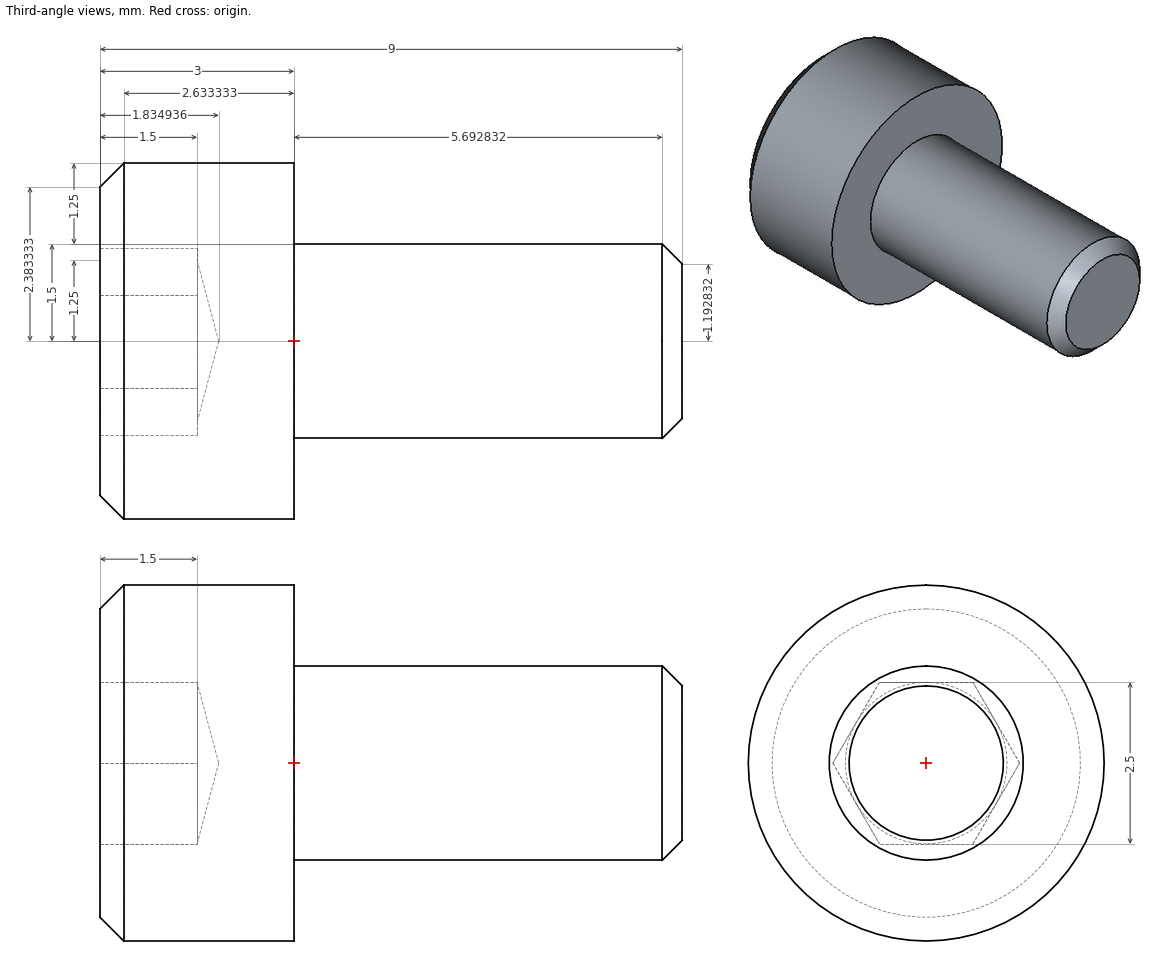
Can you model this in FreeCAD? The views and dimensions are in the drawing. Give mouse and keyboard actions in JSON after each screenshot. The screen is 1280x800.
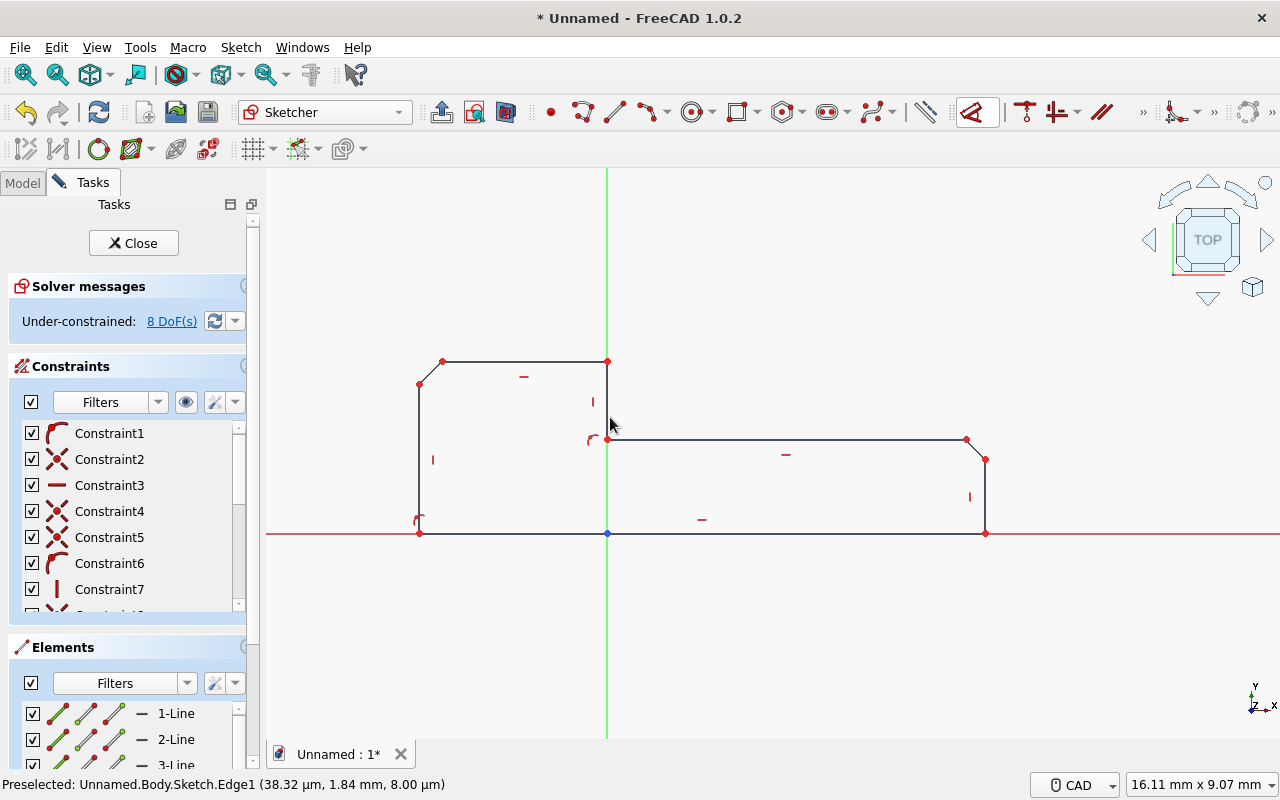
{"action": "left_click", "coordinate": [589, 534]}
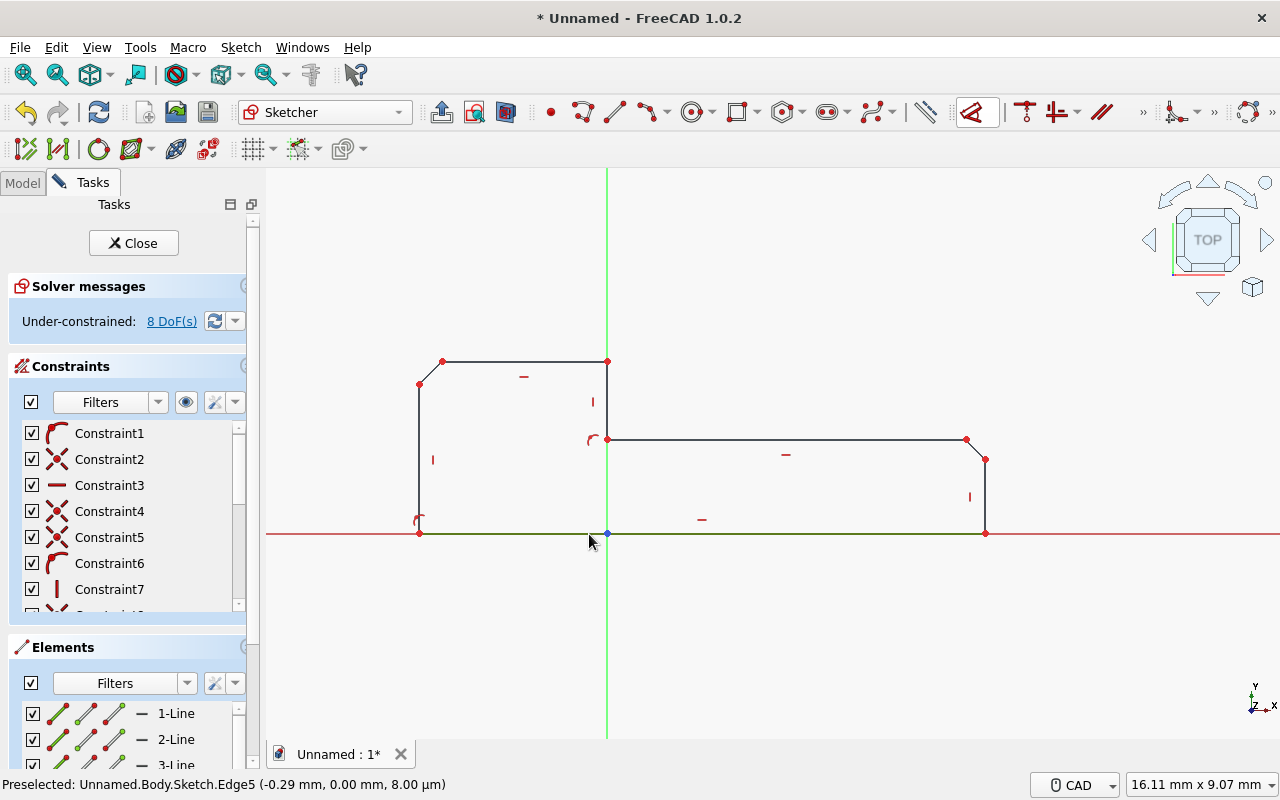
{"action": "left_click", "coordinate": [994, 112]}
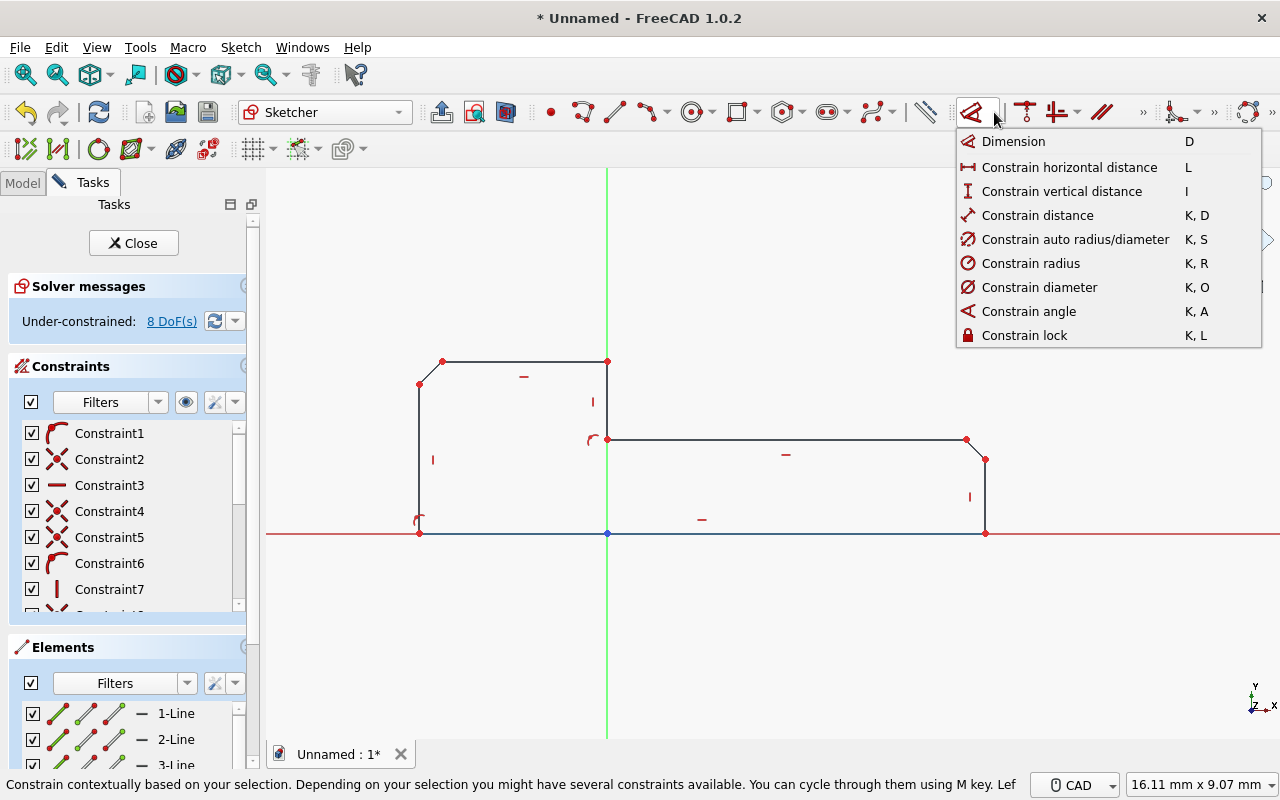
{"action": "left_click", "coordinate": [1109, 167]}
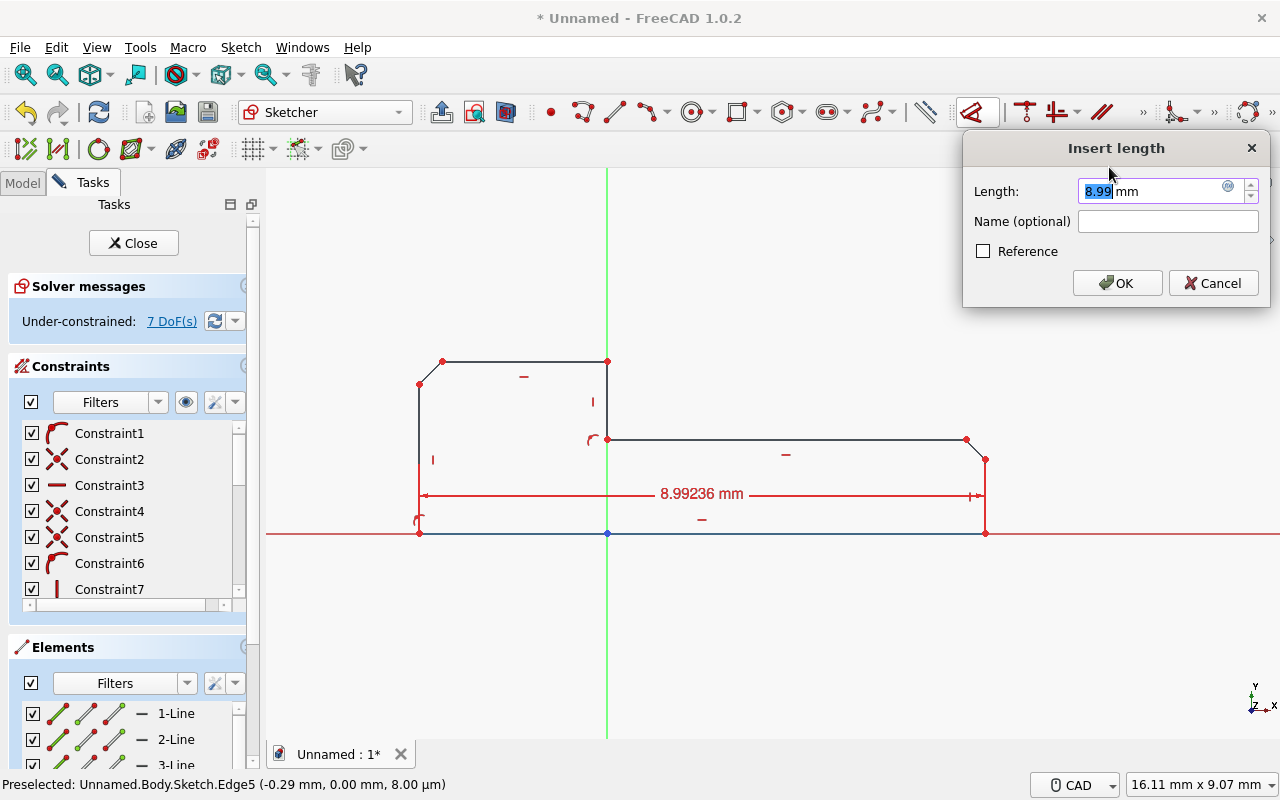
{"action": "type", "text": "9"}
{"action": "key", "text": "Return"}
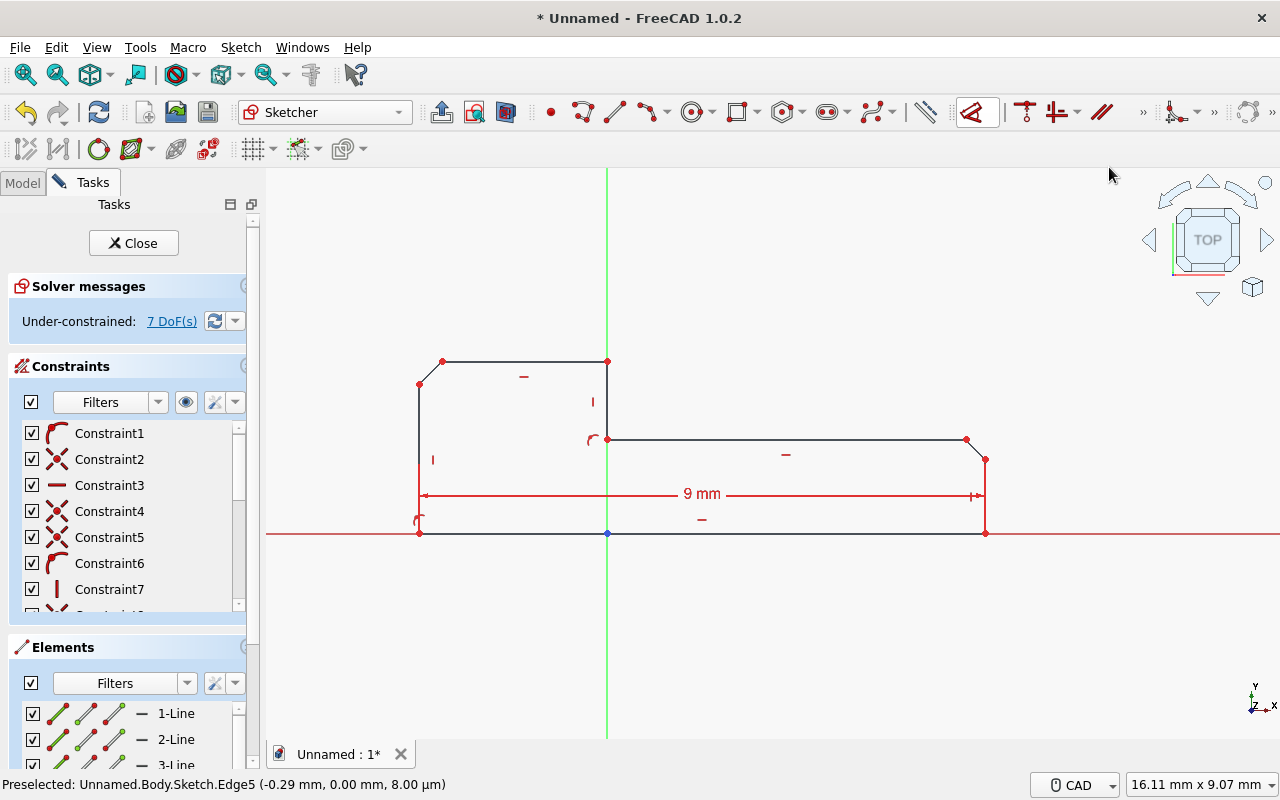
{"action": "left_click", "coordinate": [419, 385]}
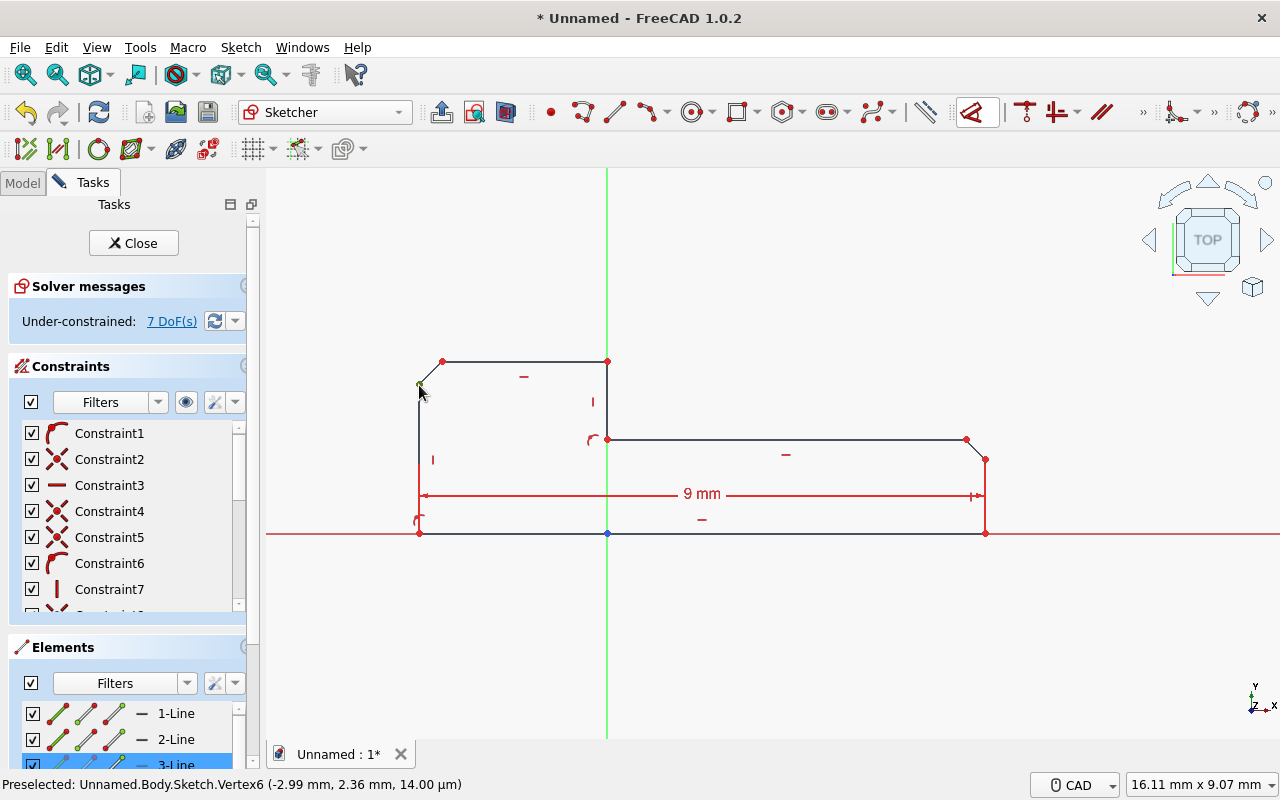
{"action": "left_click", "coordinate": [994, 112]}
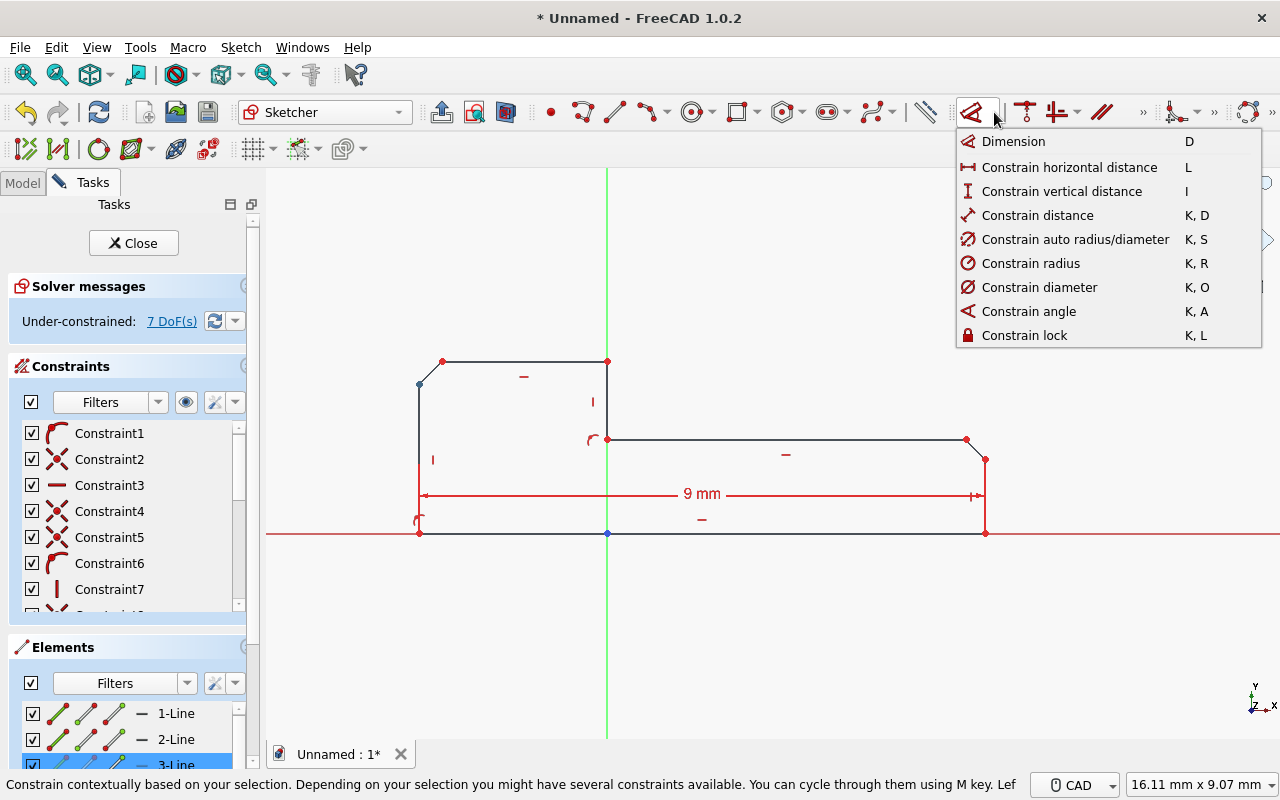
{"action": "left_click", "coordinate": [1109, 167]}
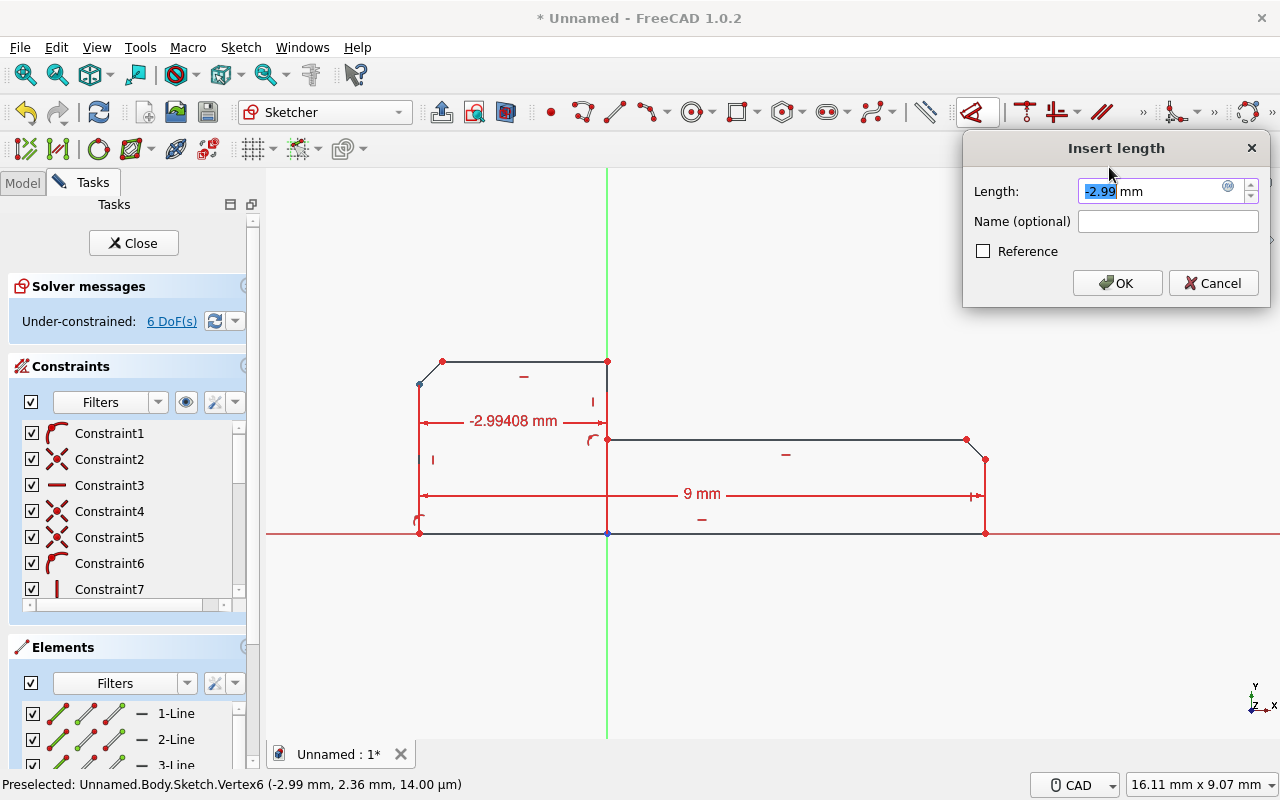
{"action": "type", "text": "-3"}
{"action": "key", "text": "Return"}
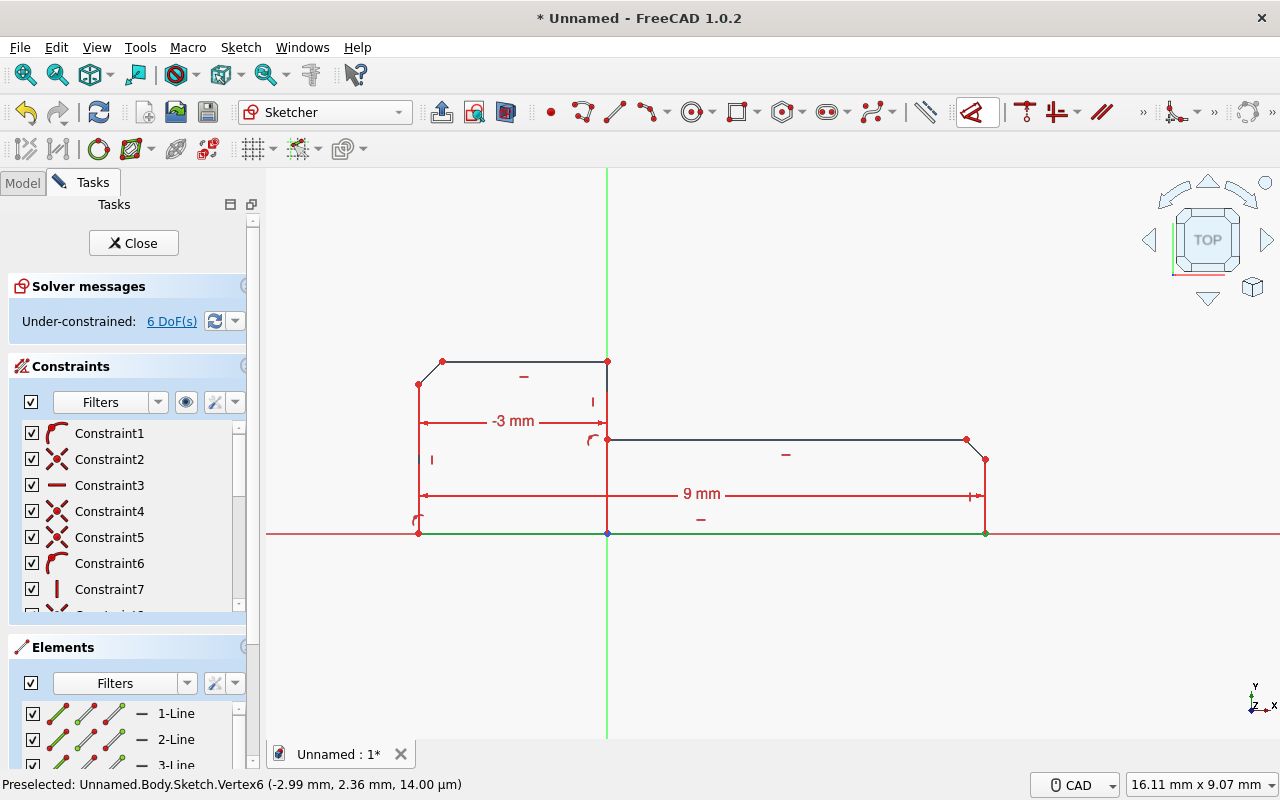
{"action": "left_click", "coordinate": [607, 417]}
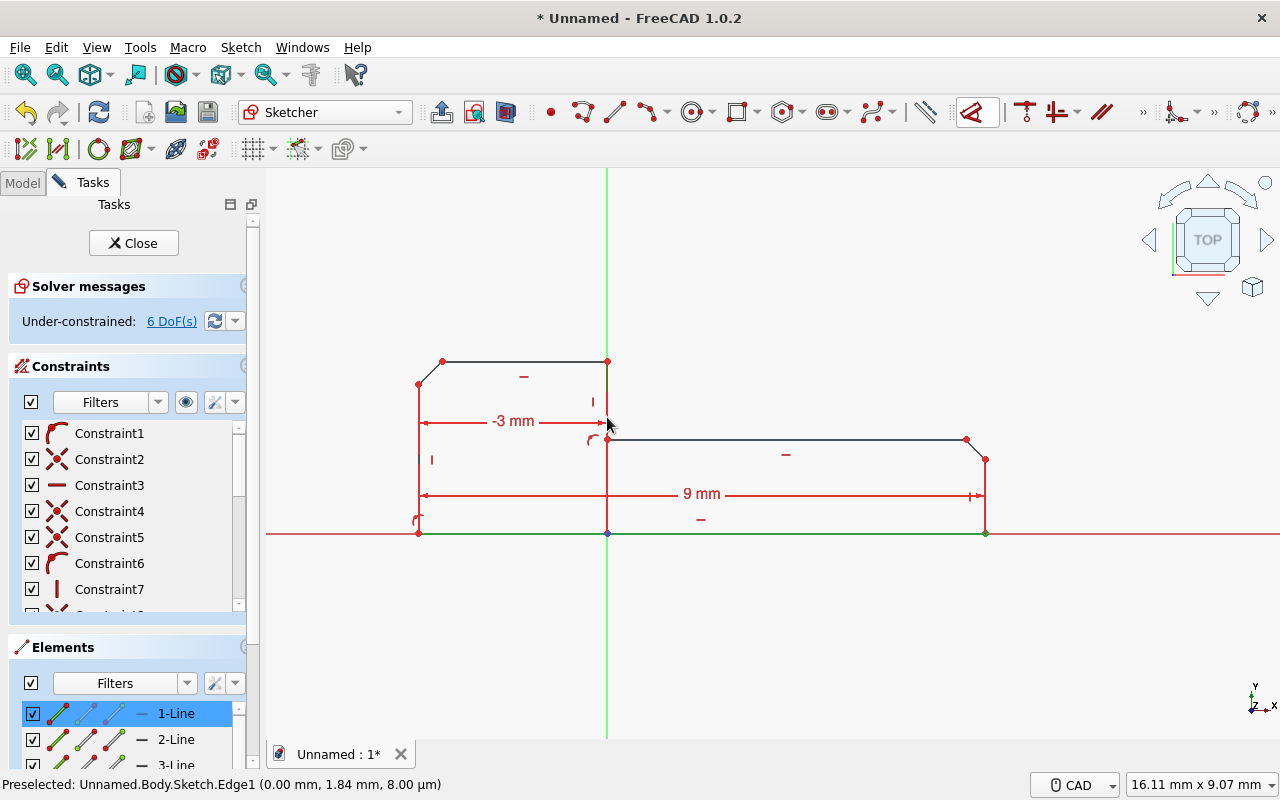
{"action": "left_click", "coordinate": [994, 112]}